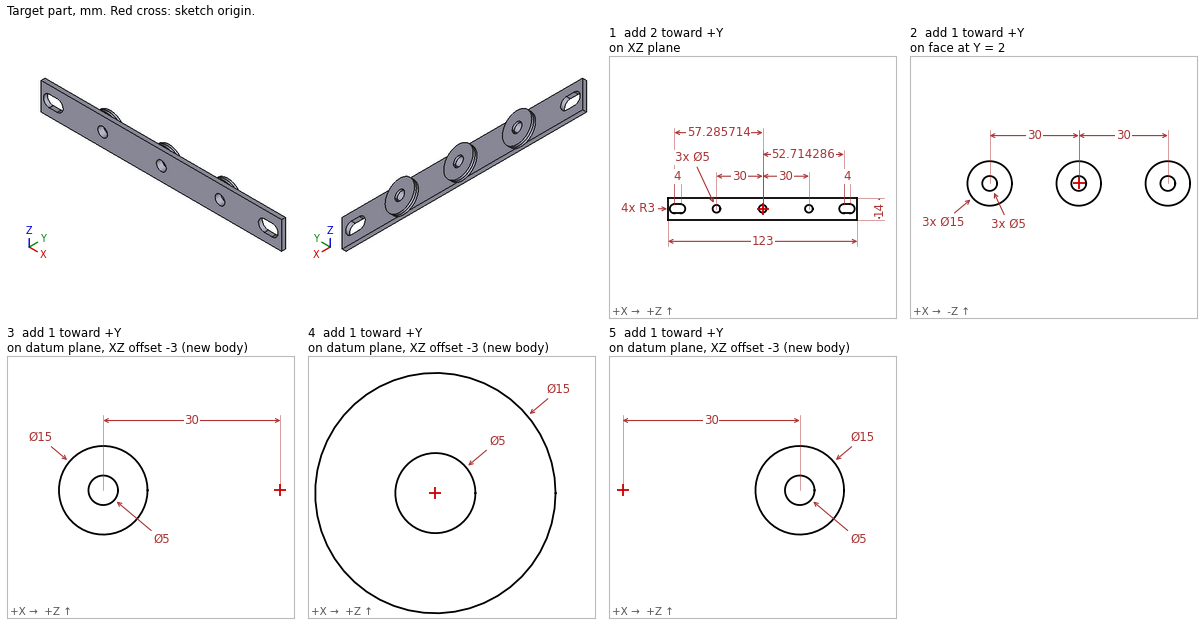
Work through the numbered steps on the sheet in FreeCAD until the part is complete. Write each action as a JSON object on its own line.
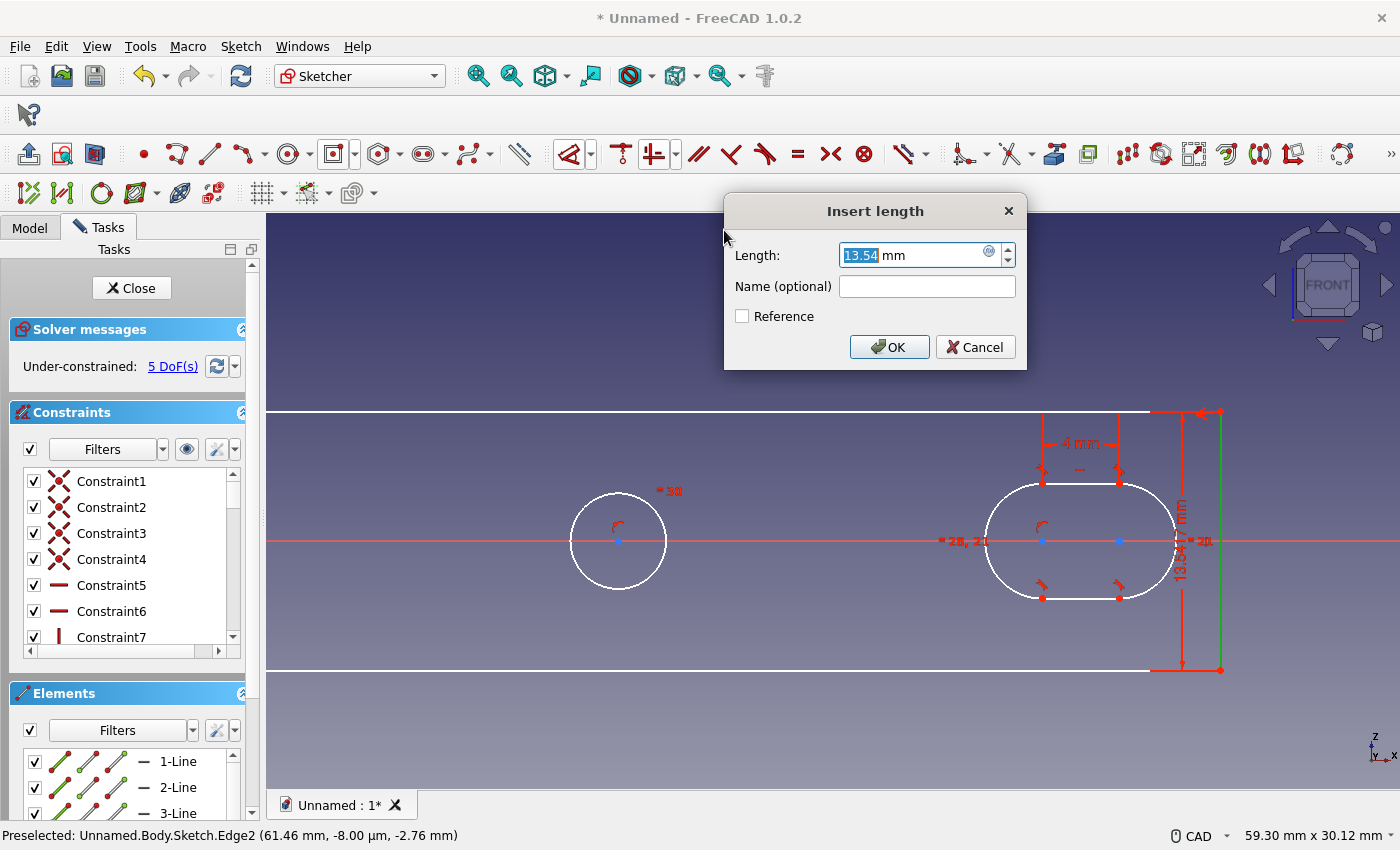
{"action": "type", "text": "14"}
{"action": "key", "text": "Return"}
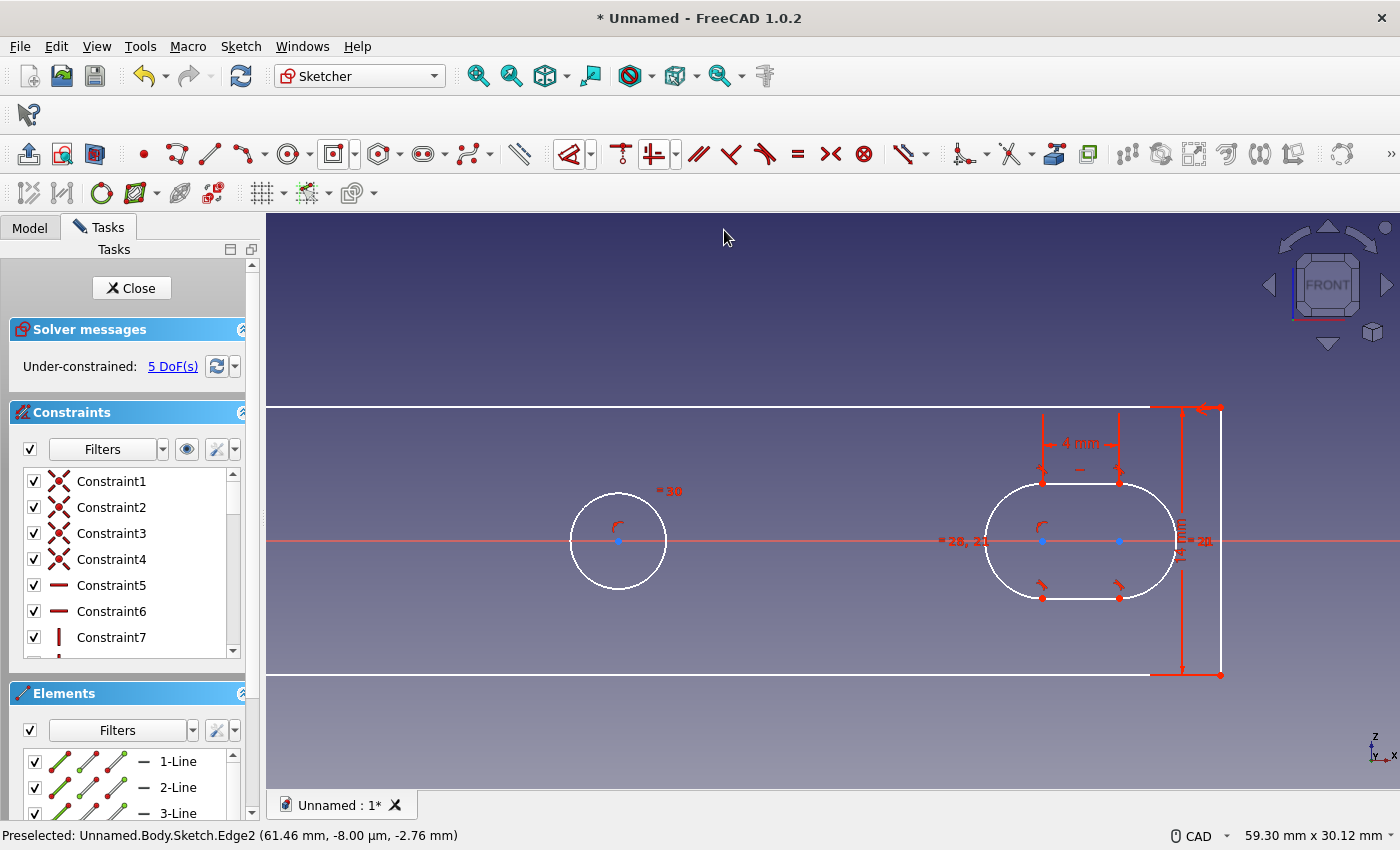
{"action": "scroll", "coordinate": [1074, 484], "scroll_direction": "down", "scroll_amount": 6}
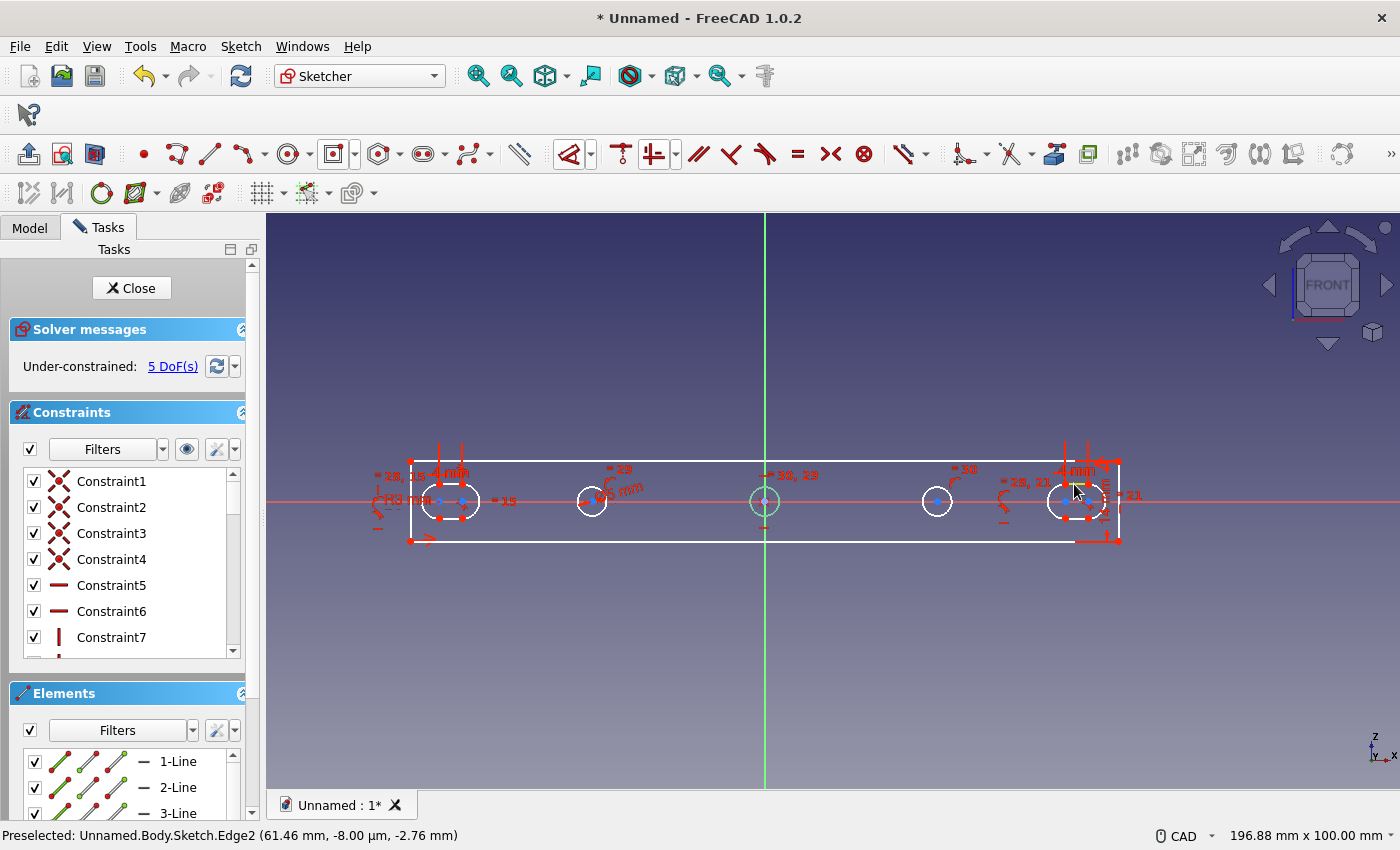
{"action": "left_click", "coordinate": [592, 502]}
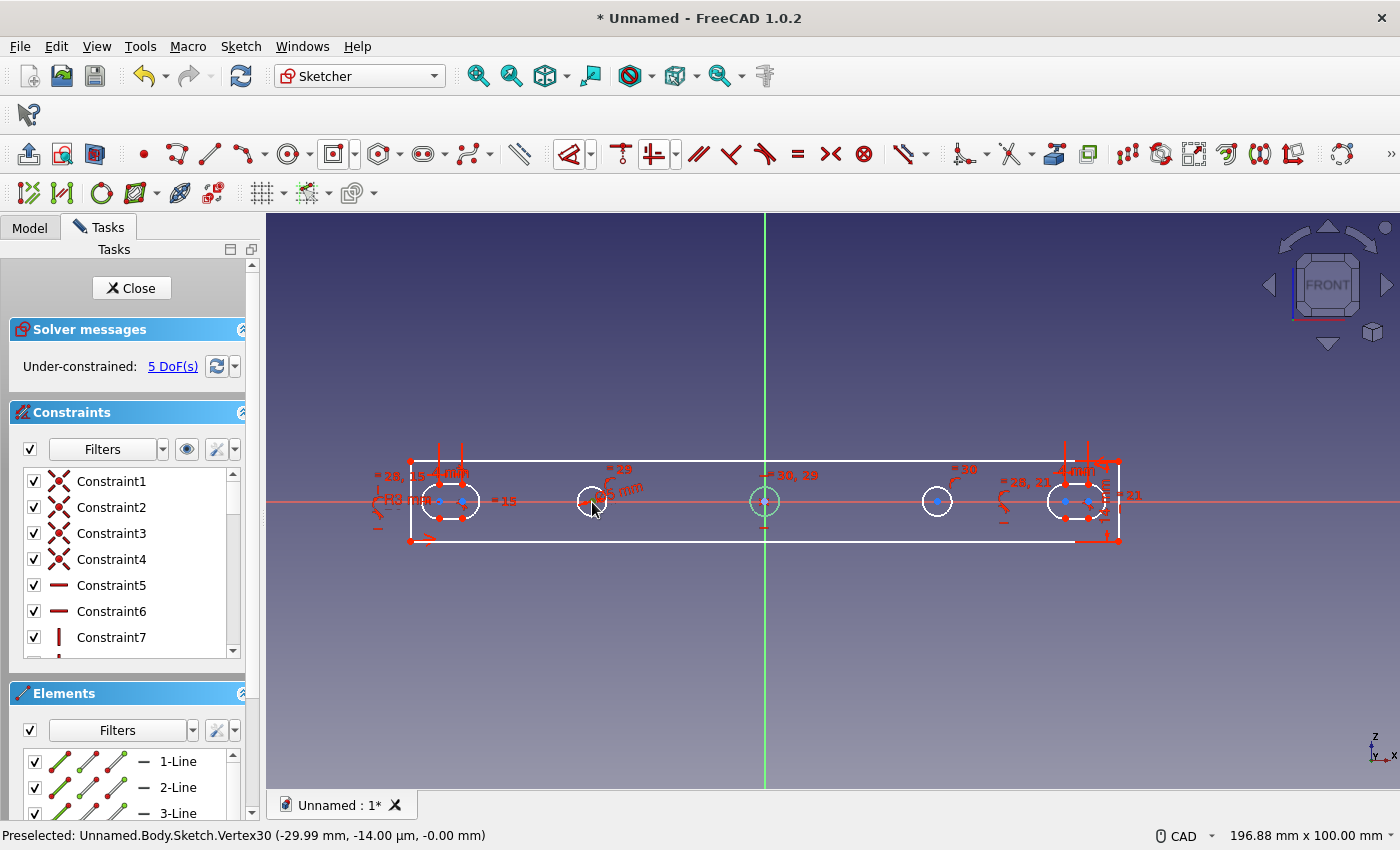
{"action": "left_click", "coordinate": [590, 154]}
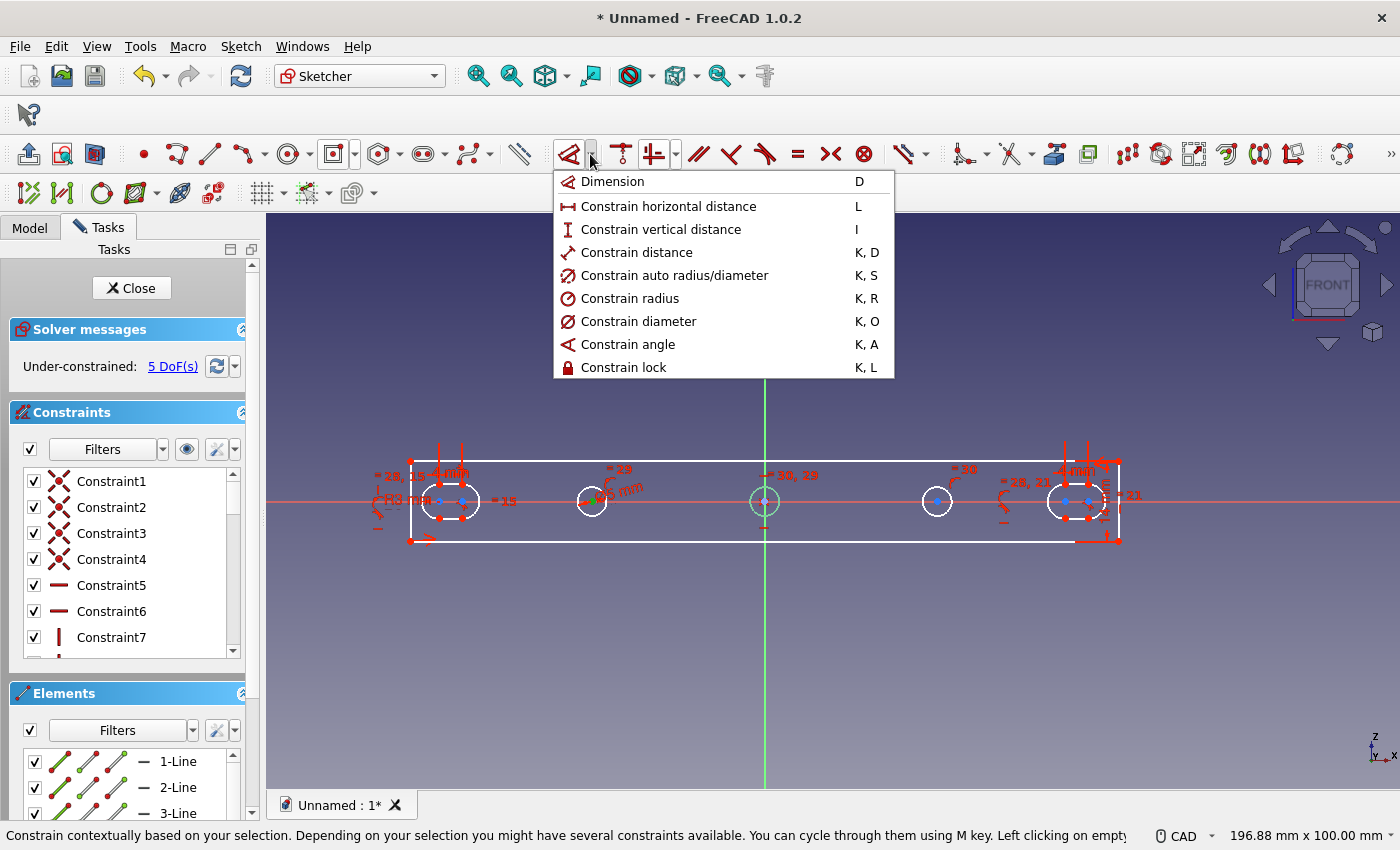
{"action": "left_click", "coordinate": [724, 206]}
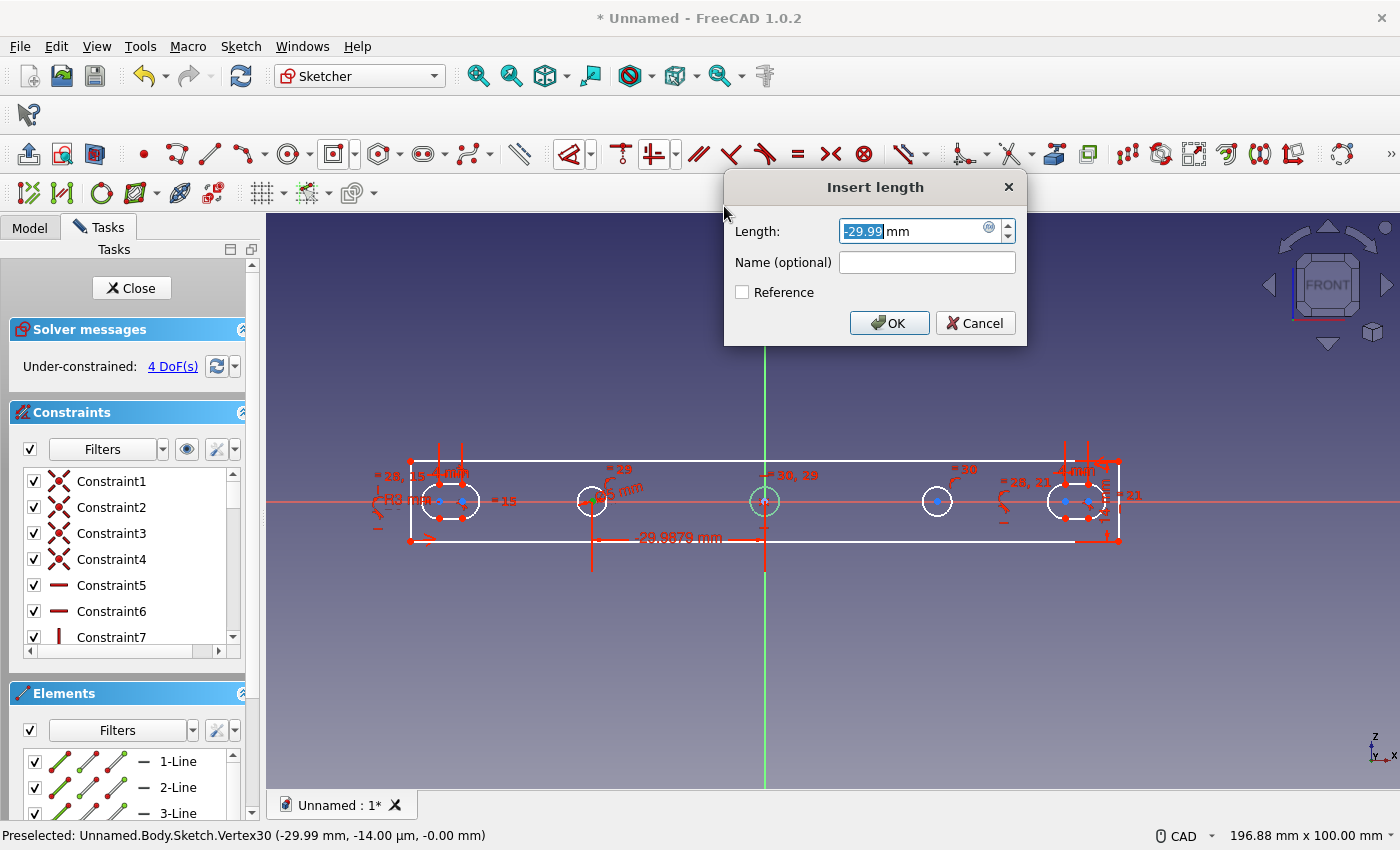
{"action": "type", "text": "-30"}
{"action": "key", "text": "Return"}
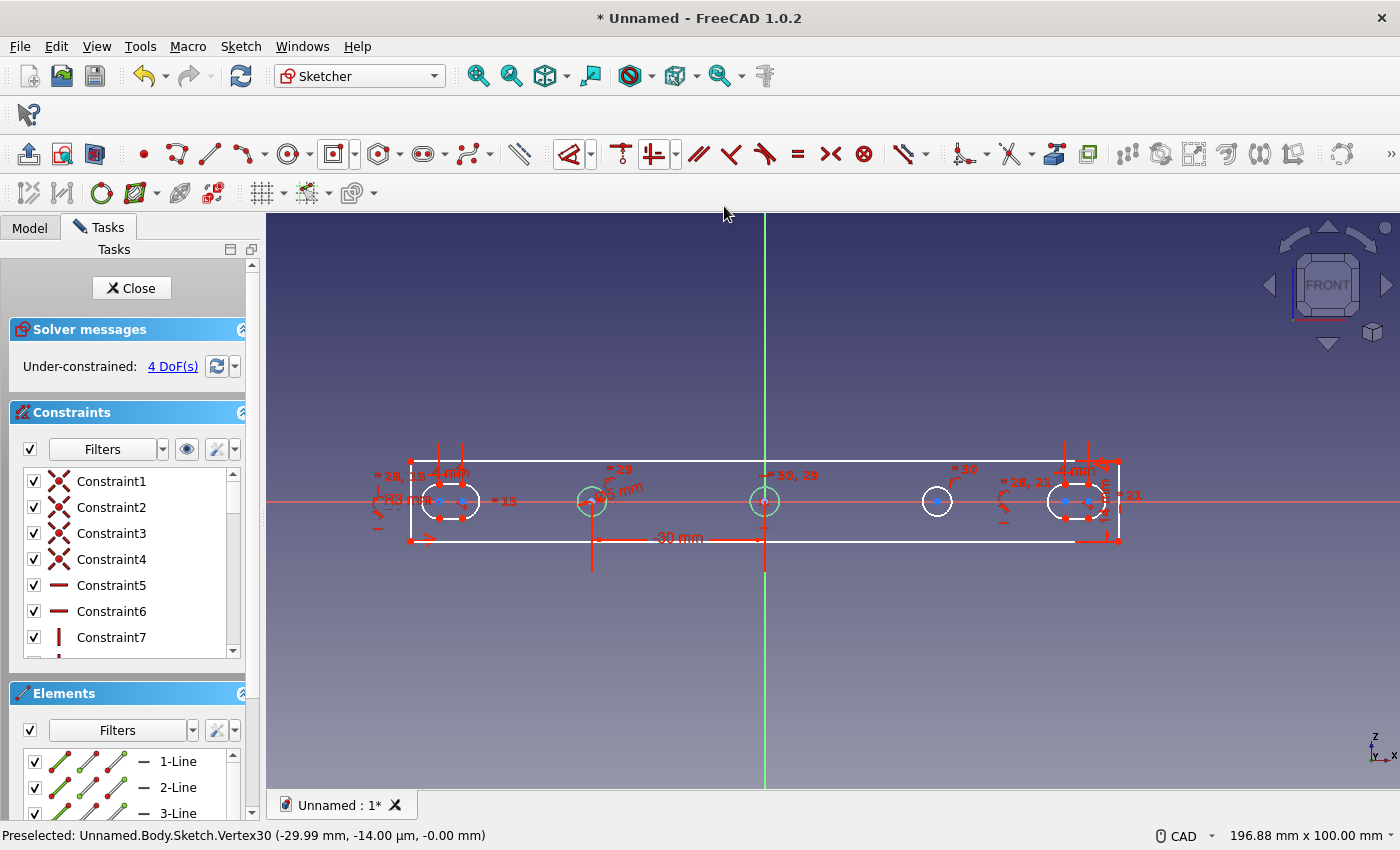
{"action": "left_click", "coordinate": [937, 502]}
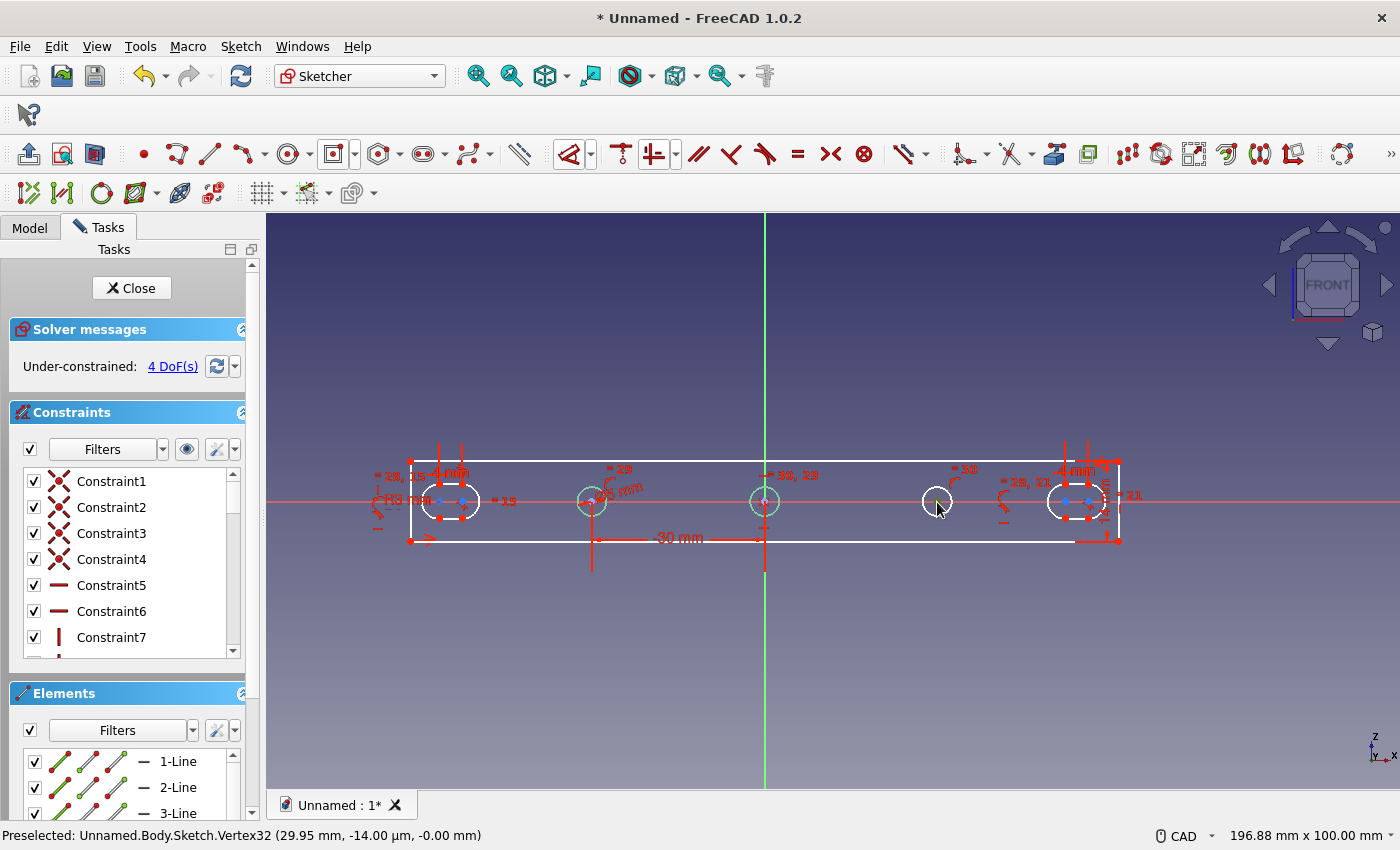
{"action": "left_click", "coordinate": [590, 154]}